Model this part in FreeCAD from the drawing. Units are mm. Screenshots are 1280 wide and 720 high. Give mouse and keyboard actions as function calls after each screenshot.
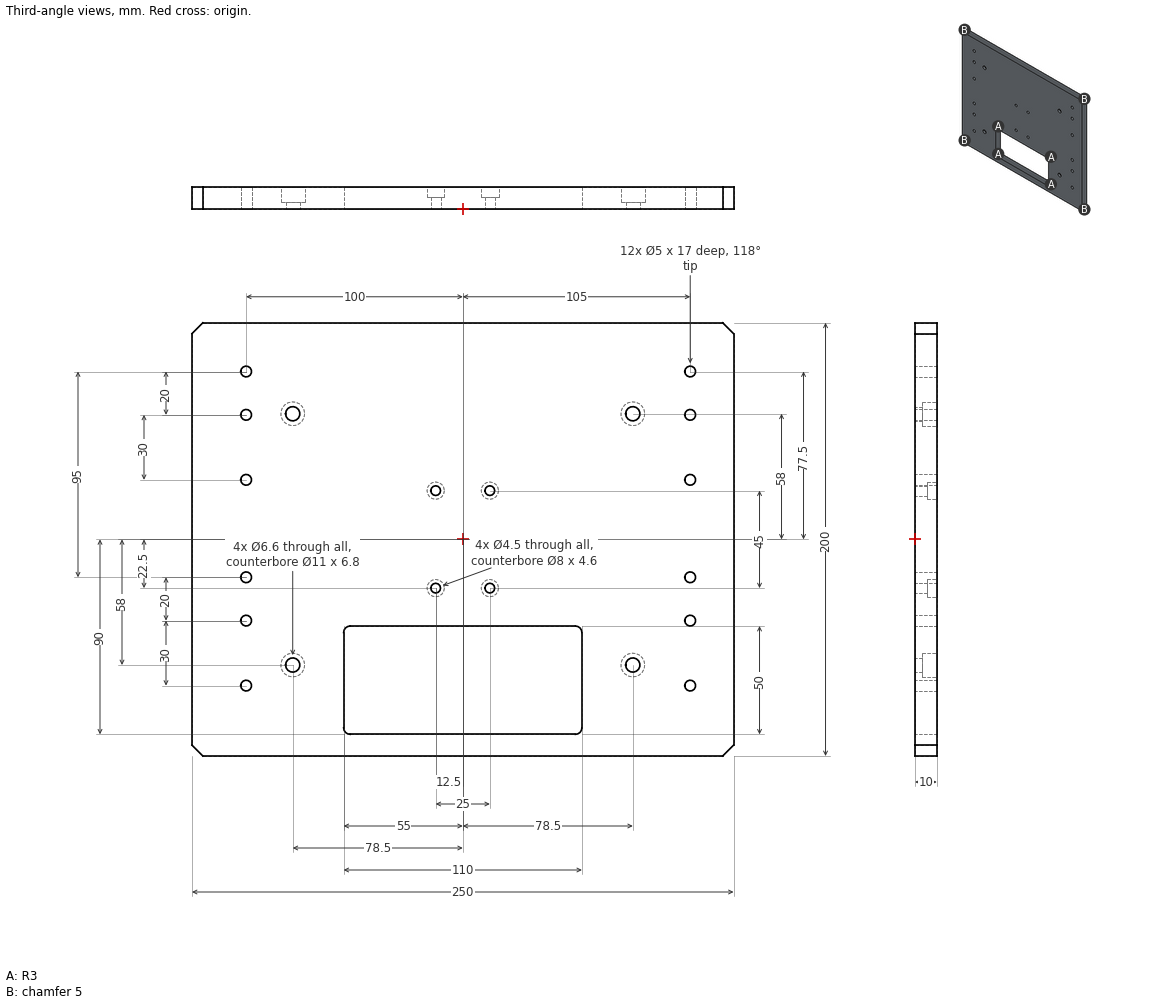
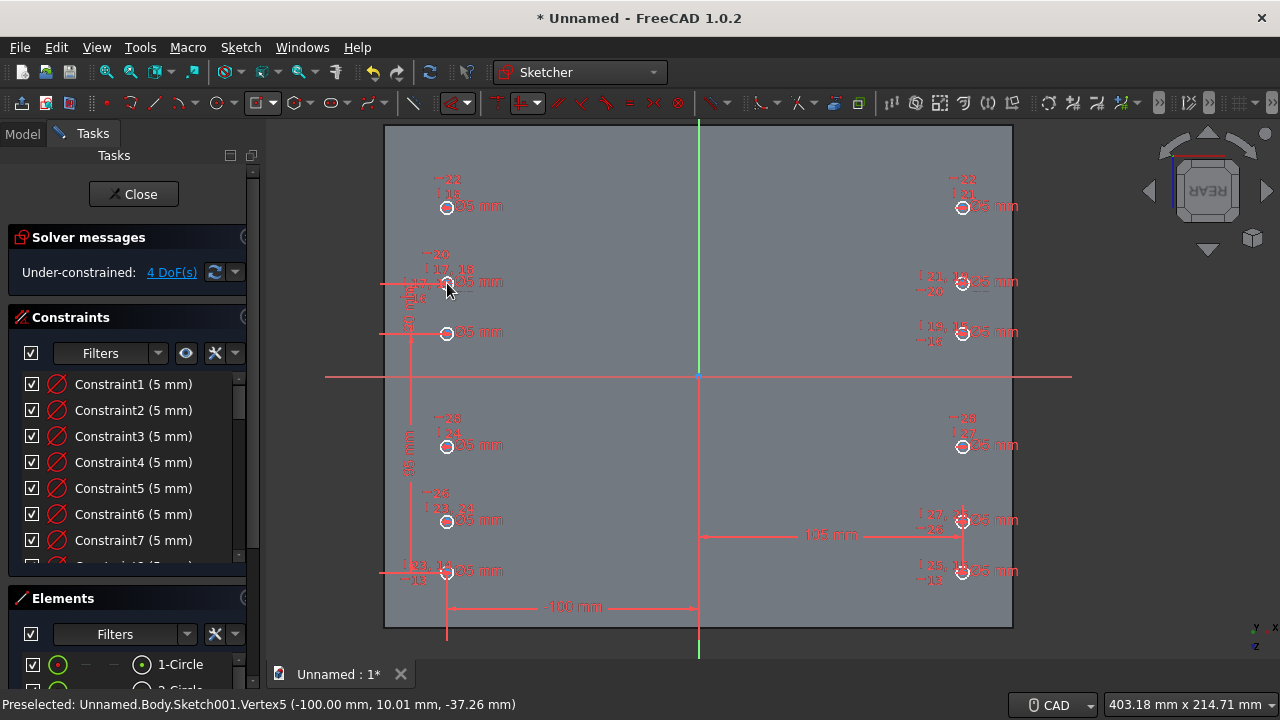
click(447, 284)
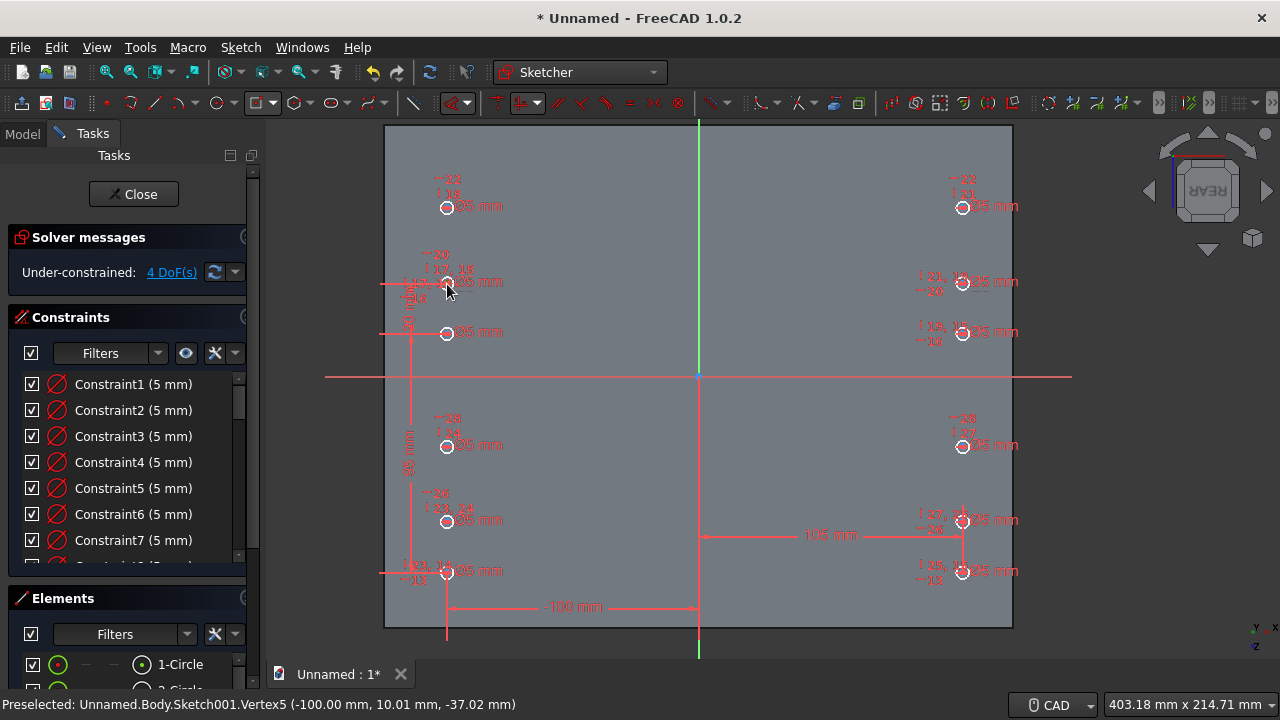
click(447, 208)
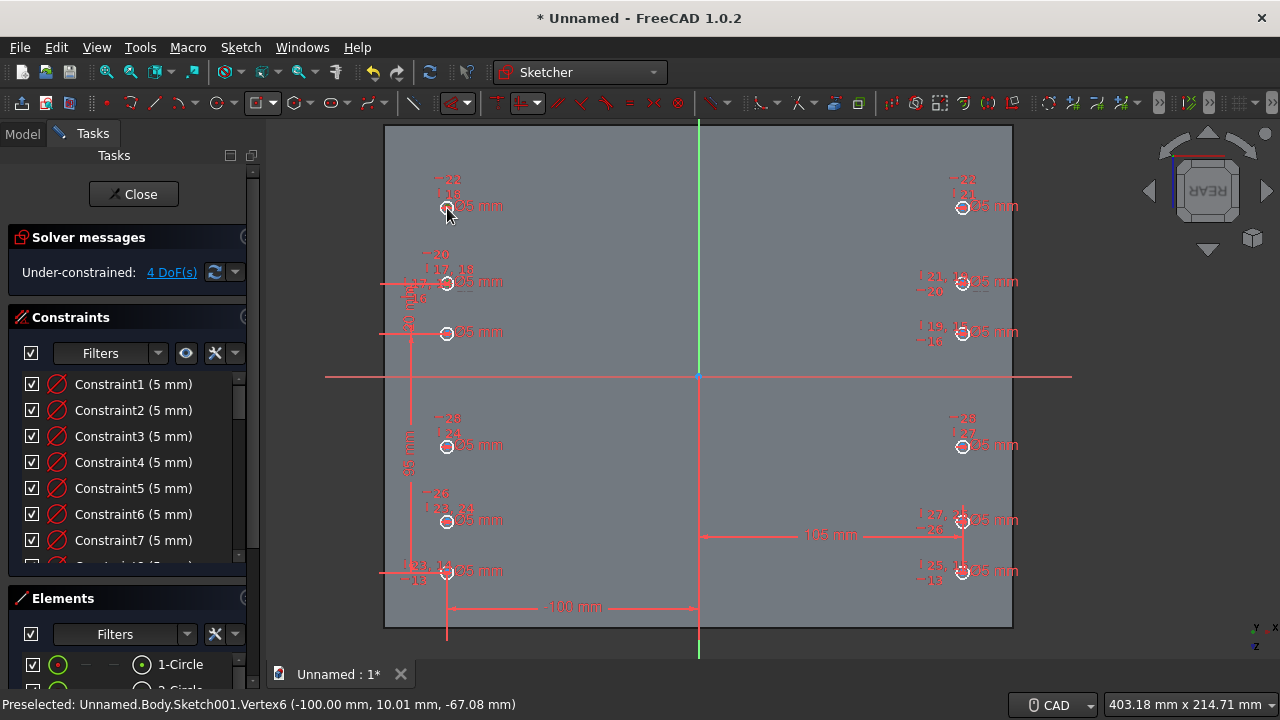
click(470, 104)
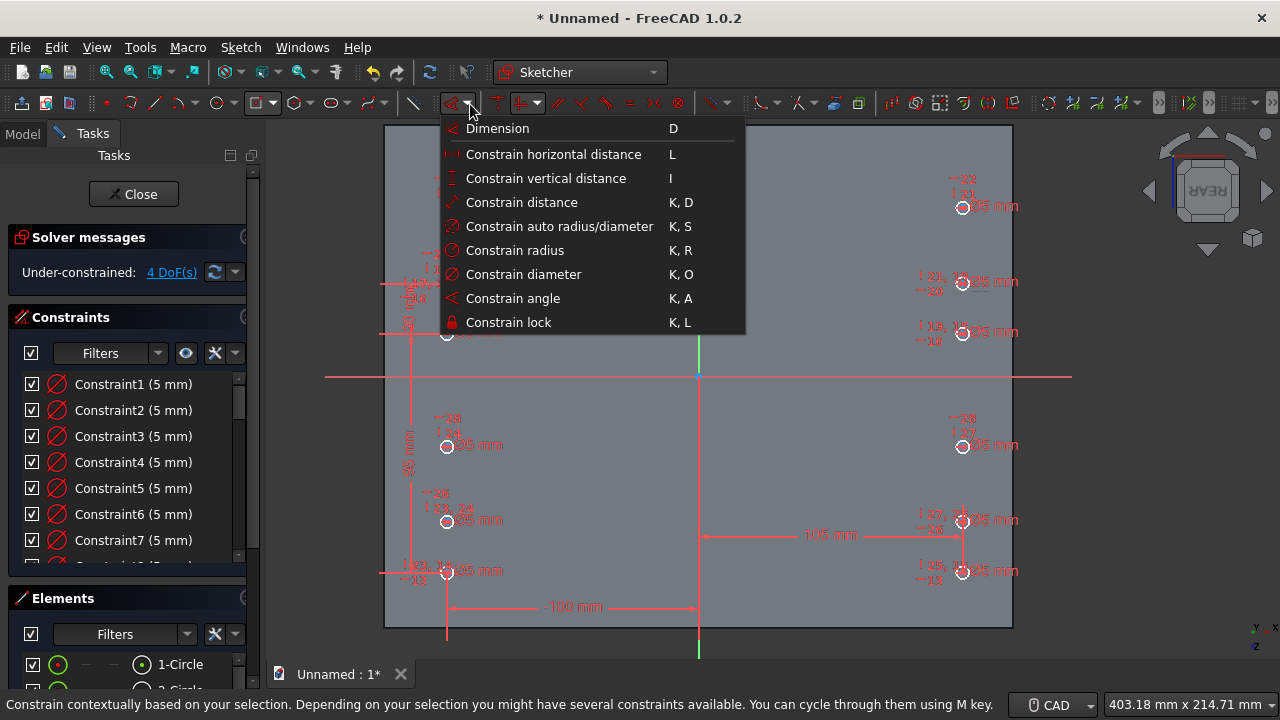
click(593, 178)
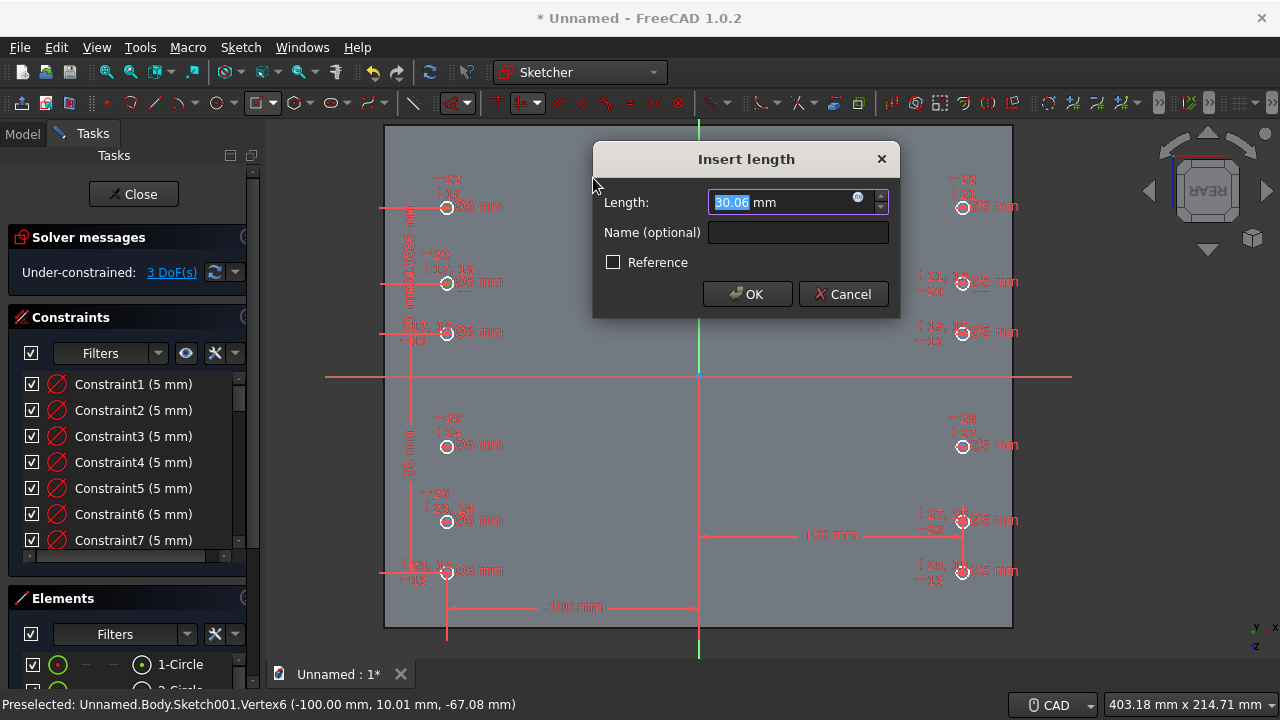
text(30)
key(Return)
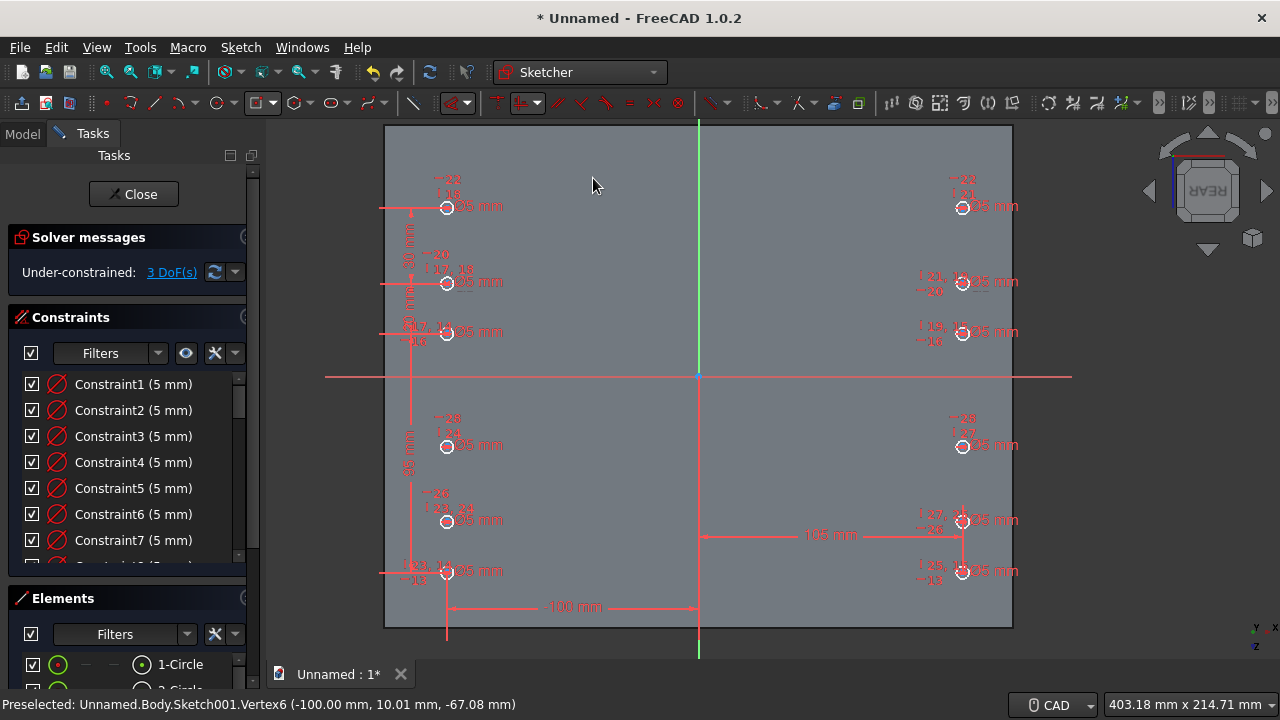
click(447, 573)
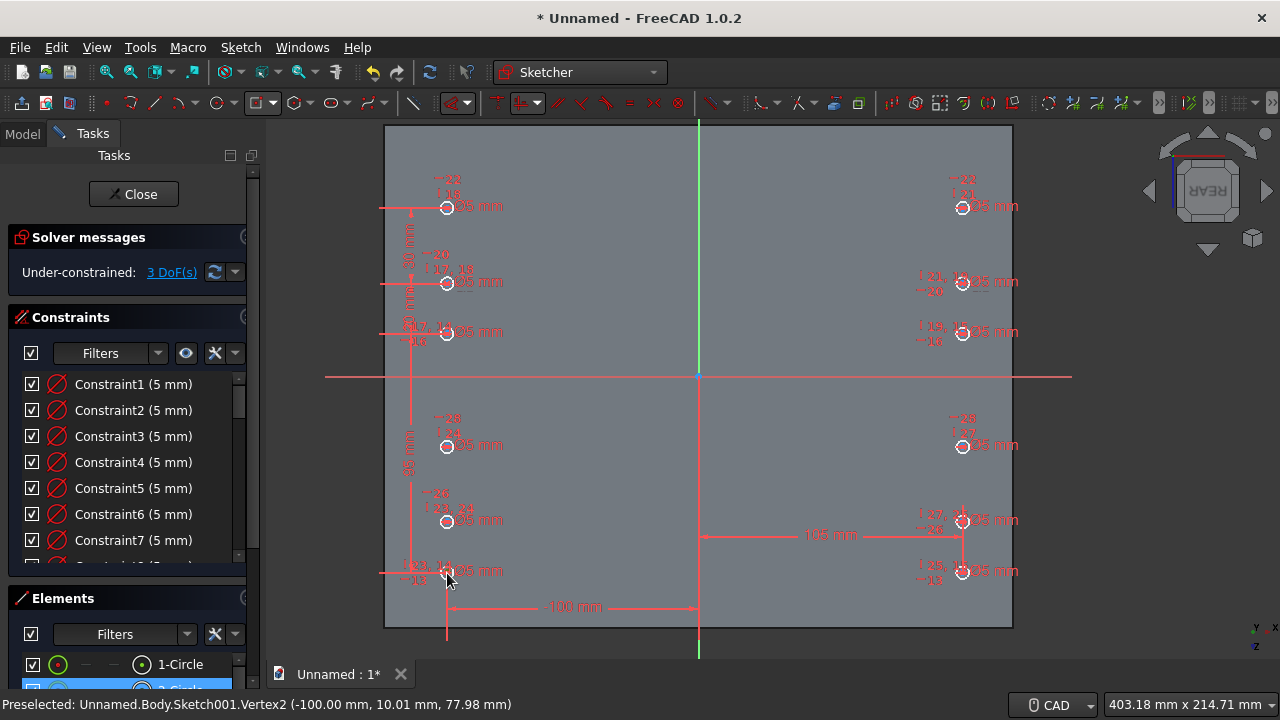
click(447, 522)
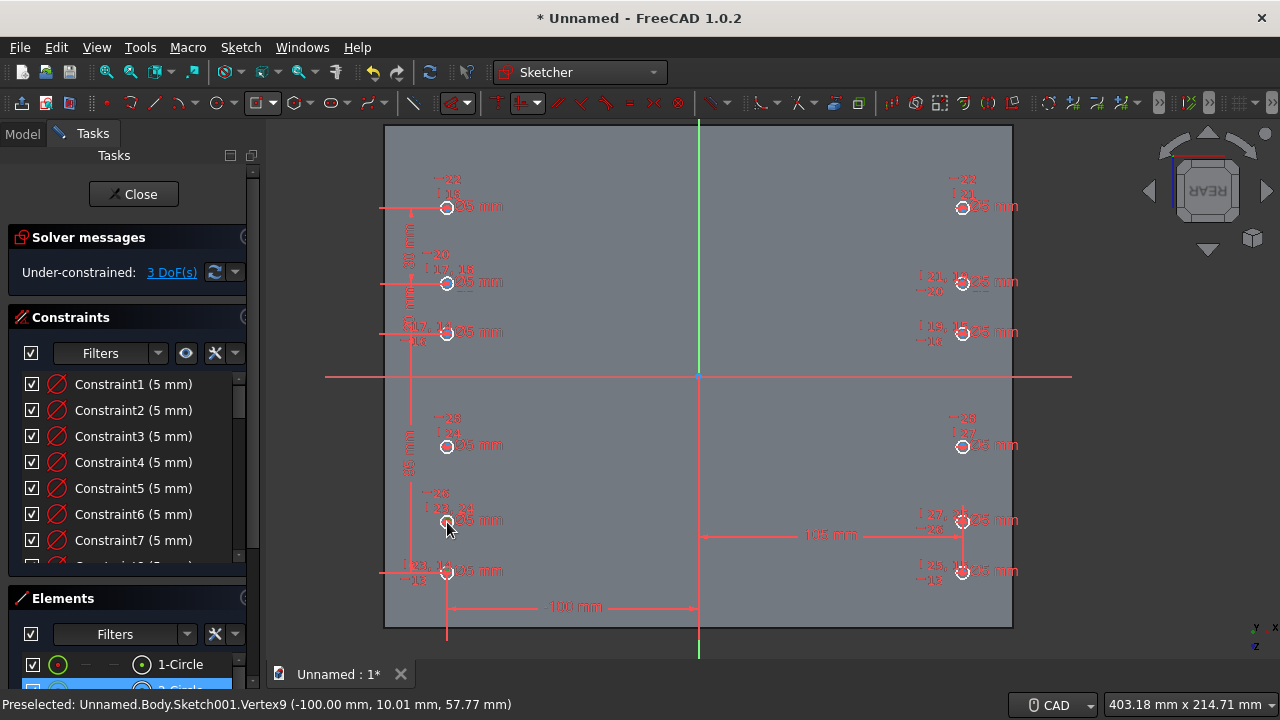
click(470, 104)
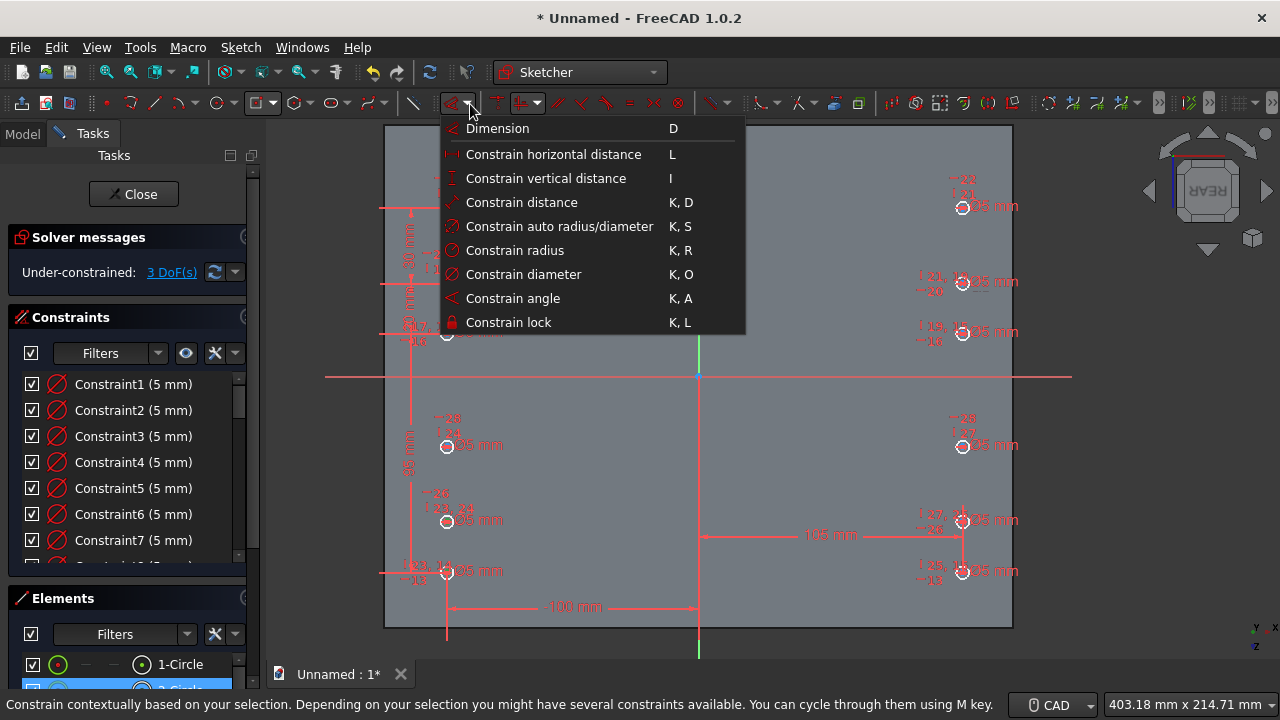
click(593, 178)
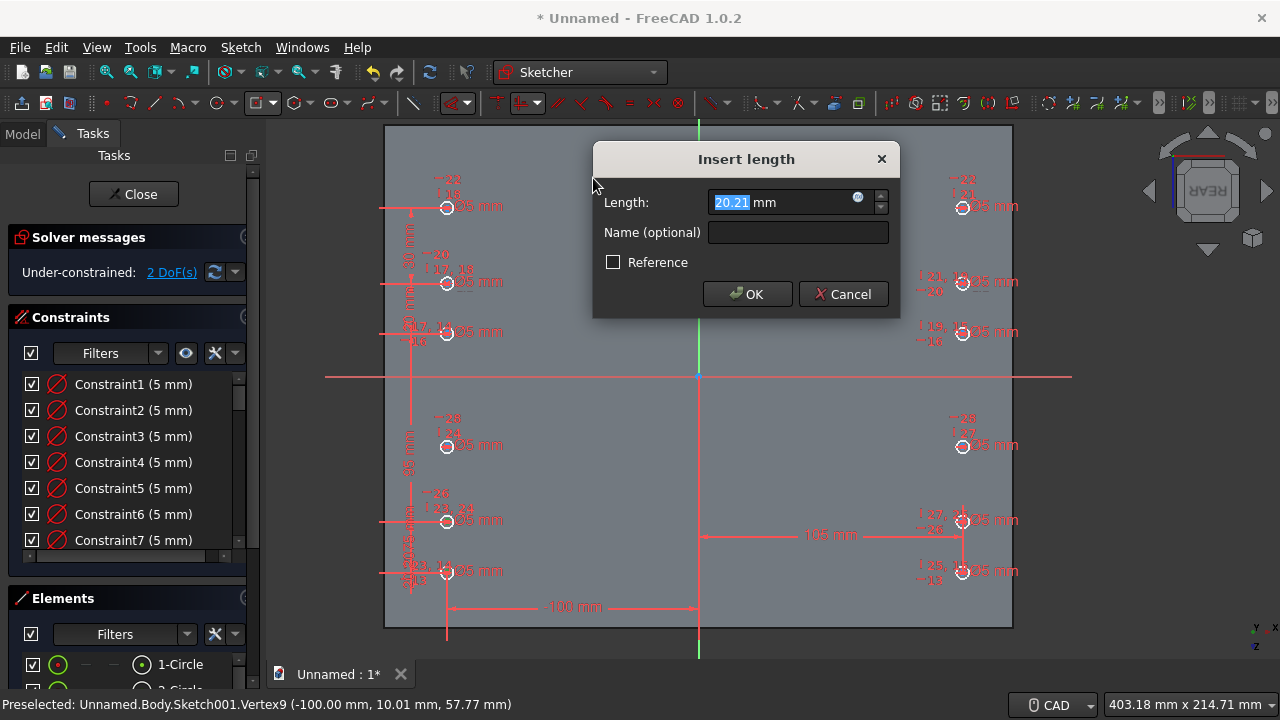
text(20)
key(Return)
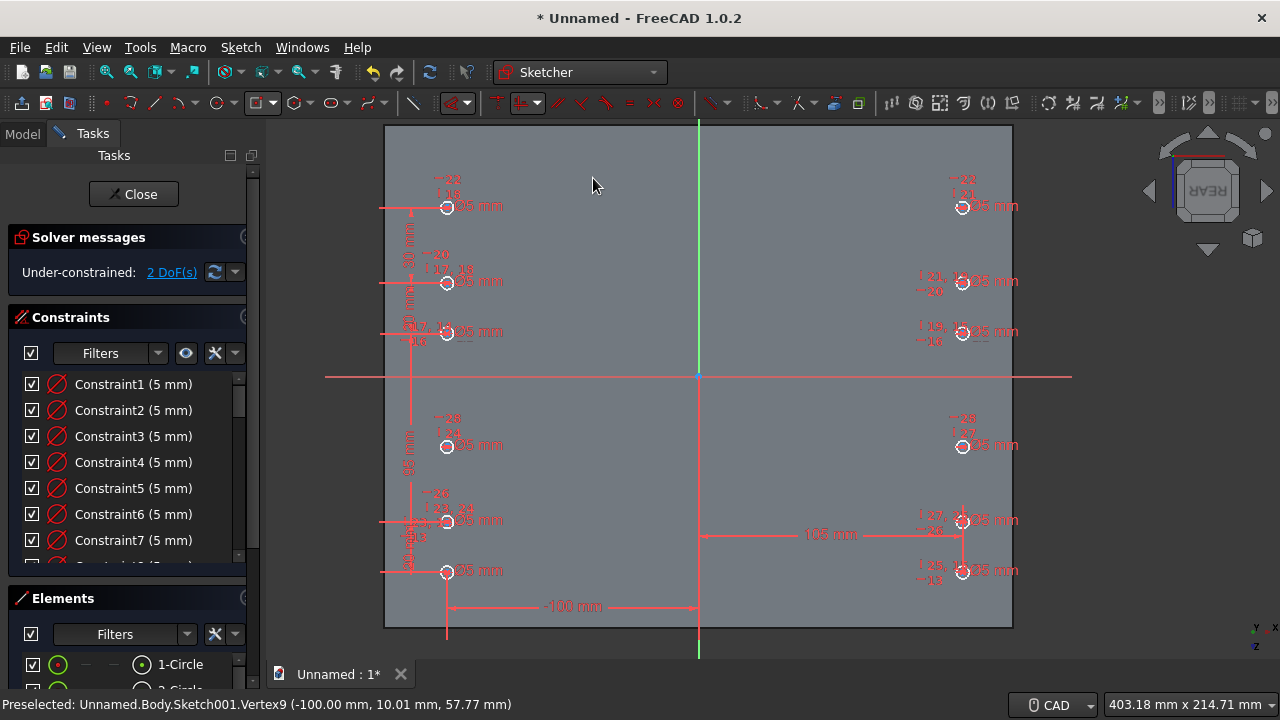
click(447, 522)